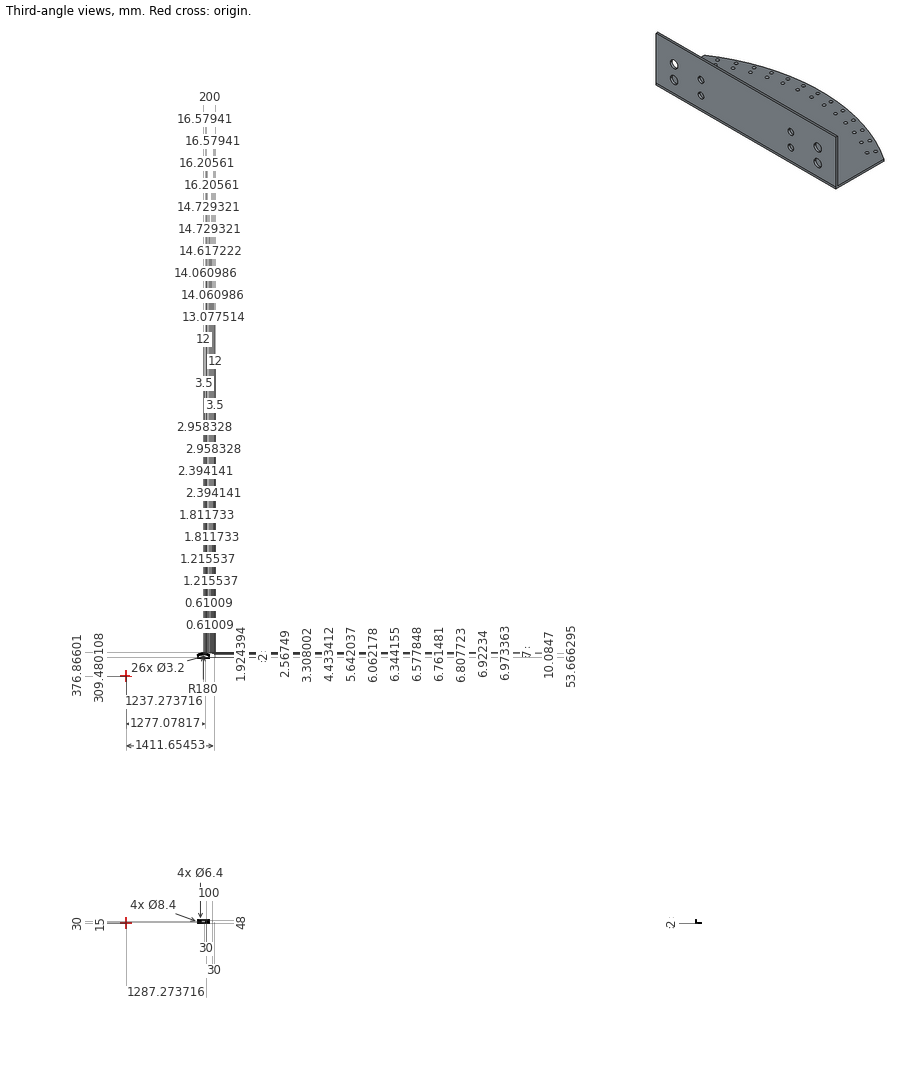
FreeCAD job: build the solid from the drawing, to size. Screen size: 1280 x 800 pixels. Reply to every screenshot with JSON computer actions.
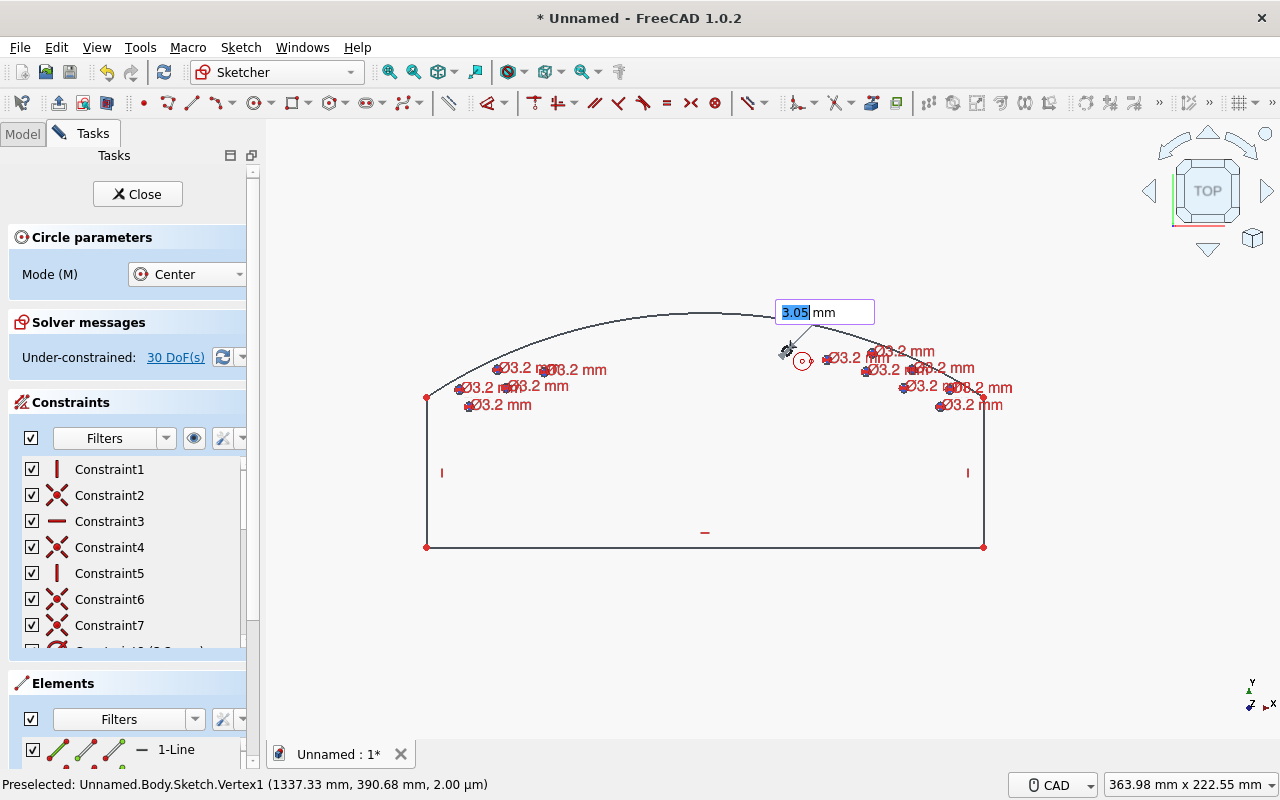
{"action": "type", "text": "3.2"}
{"action": "key", "text": "Return"}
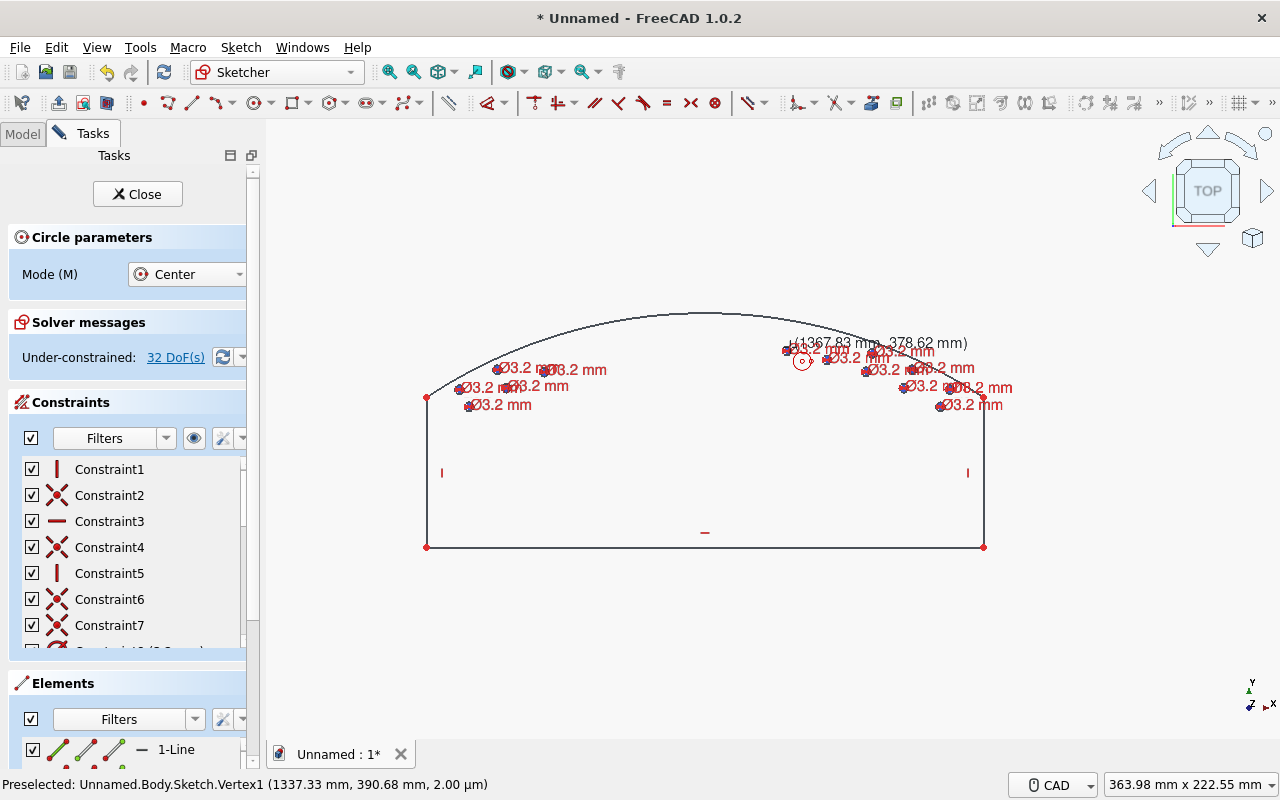
{"action": "scroll", "coordinate": [746, 345], "scroll_direction": "up", "scroll_amount": 9}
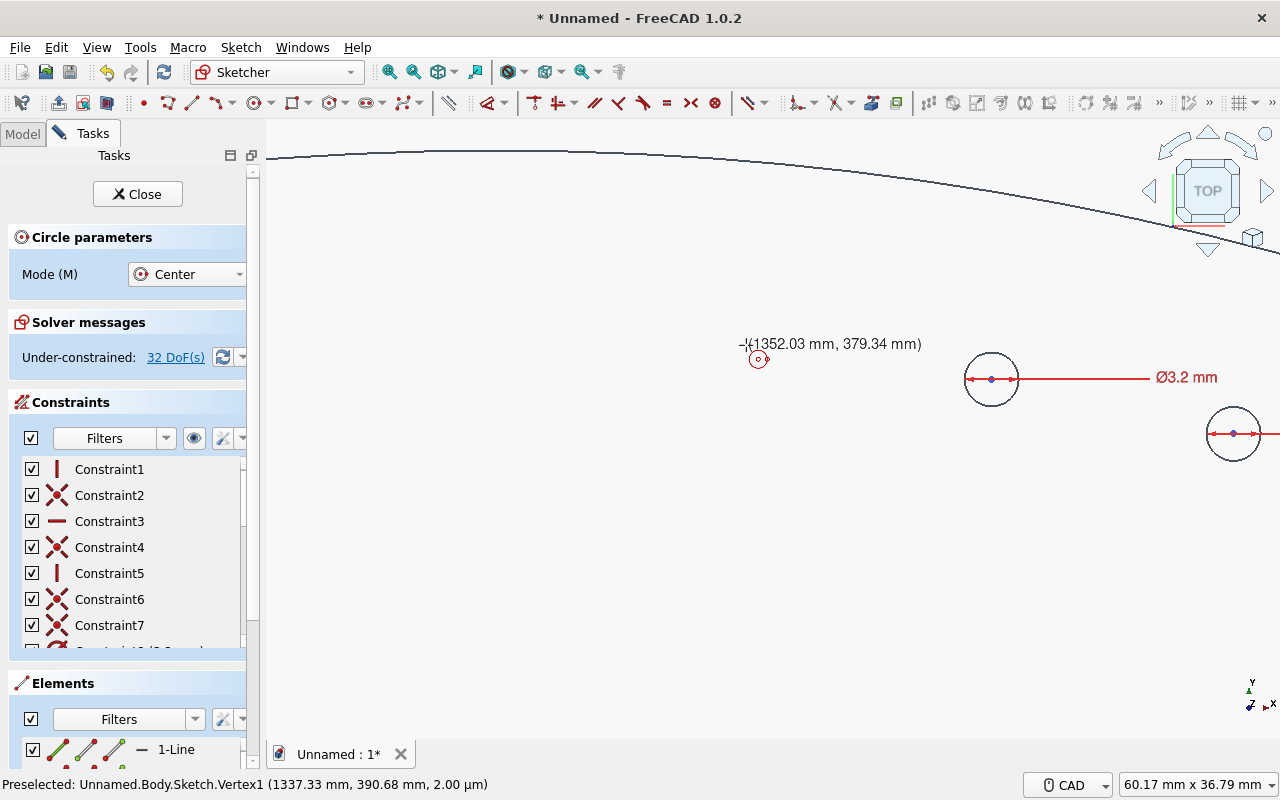
{"action": "scroll", "coordinate": [746, 345], "scroll_direction": "down", "scroll_amount": 9}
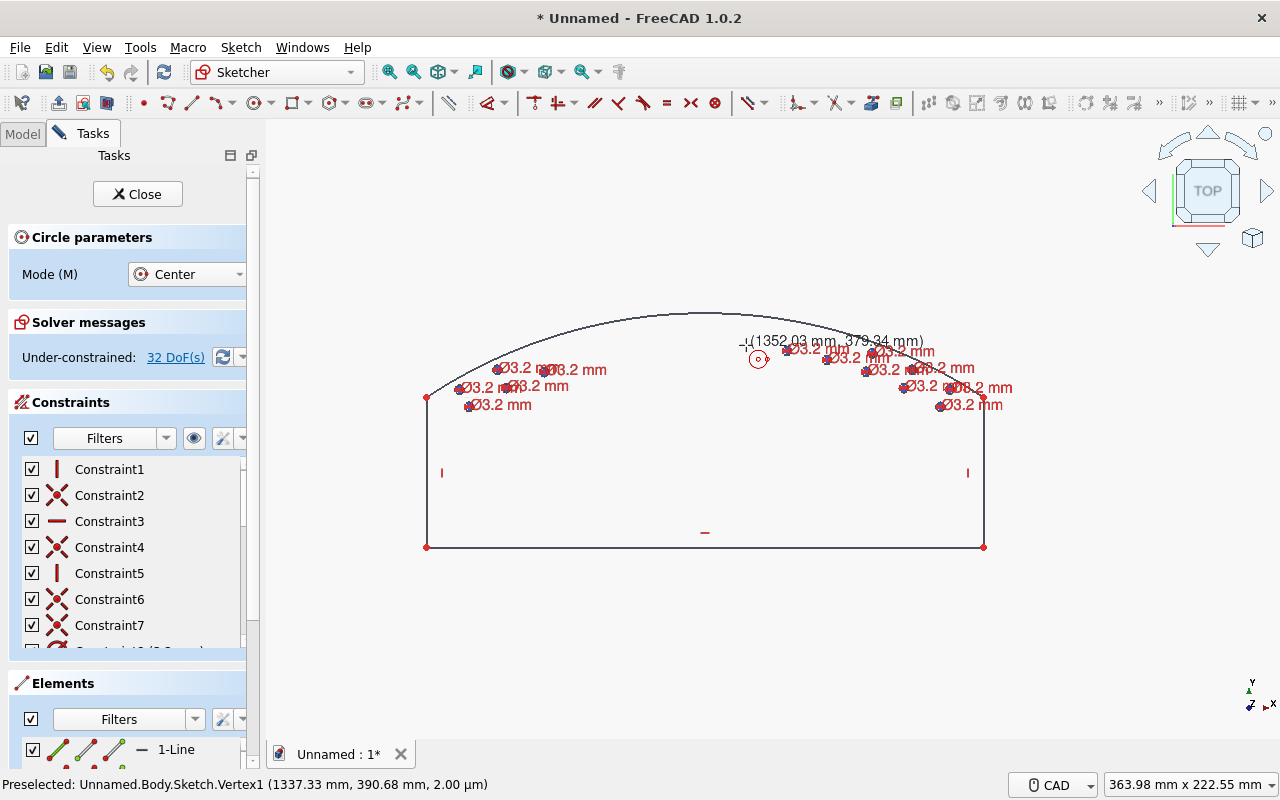
{"action": "left_click", "coordinate": [746, 345]}
{"action": "mouse_move", "coordinate": [749, 341]}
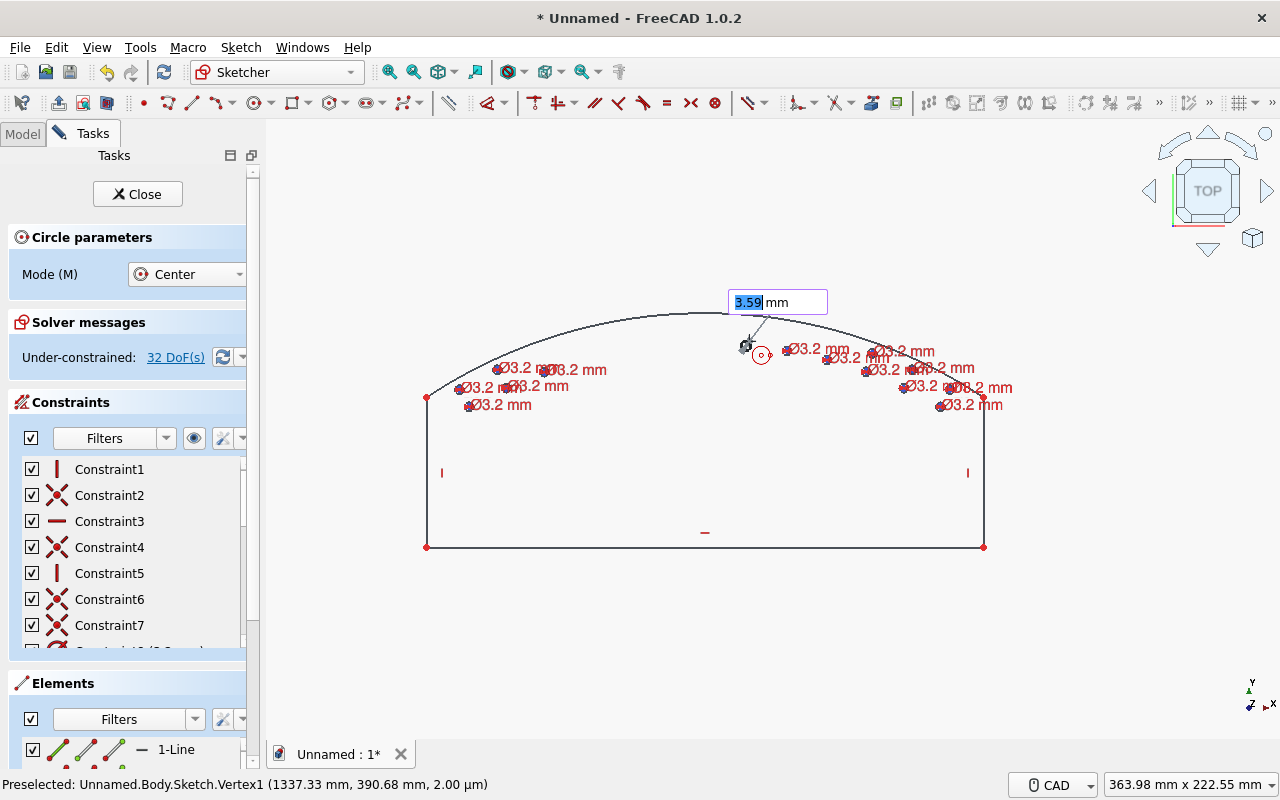
{"action": "type", "text": "3.2"}
{"action": "key", "text": "Return"}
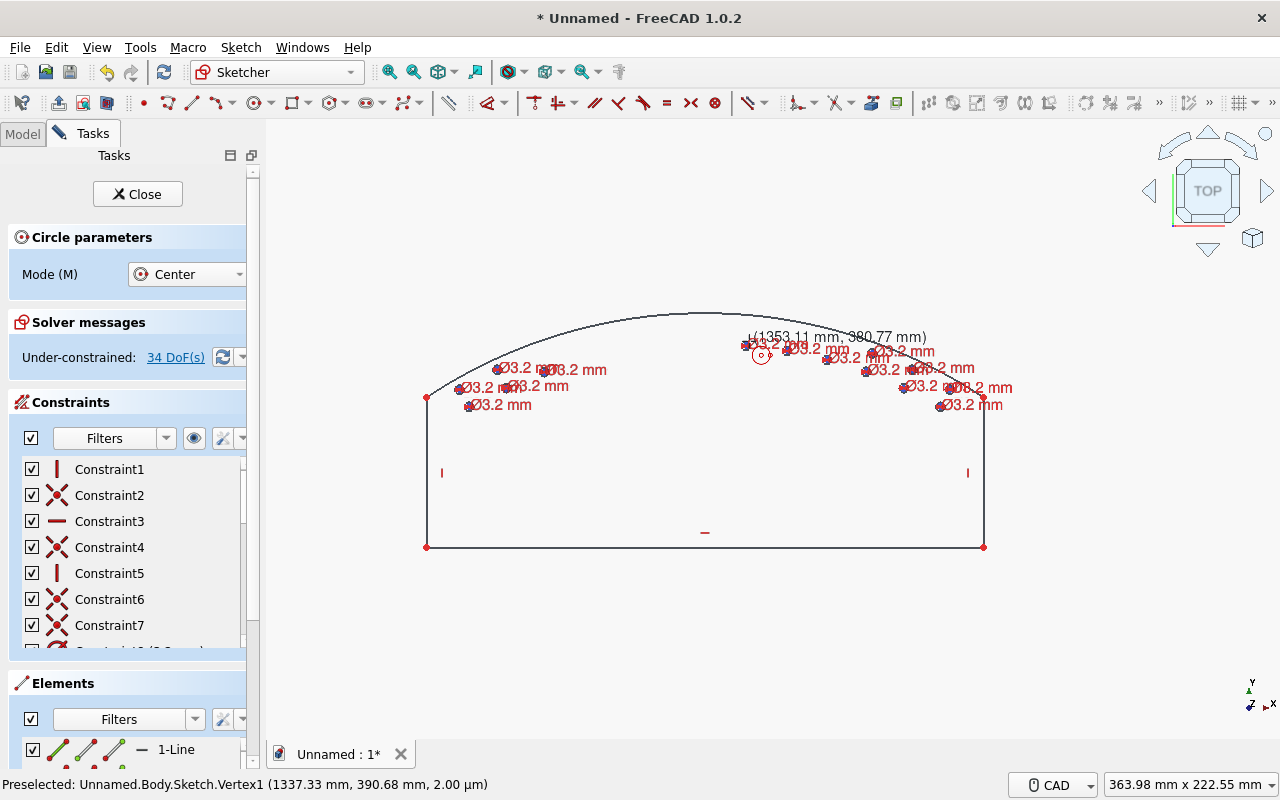
{"action": "scroll", "coordinate": [705, 343], "scroll_direction": "up", "scroll_amount": 9}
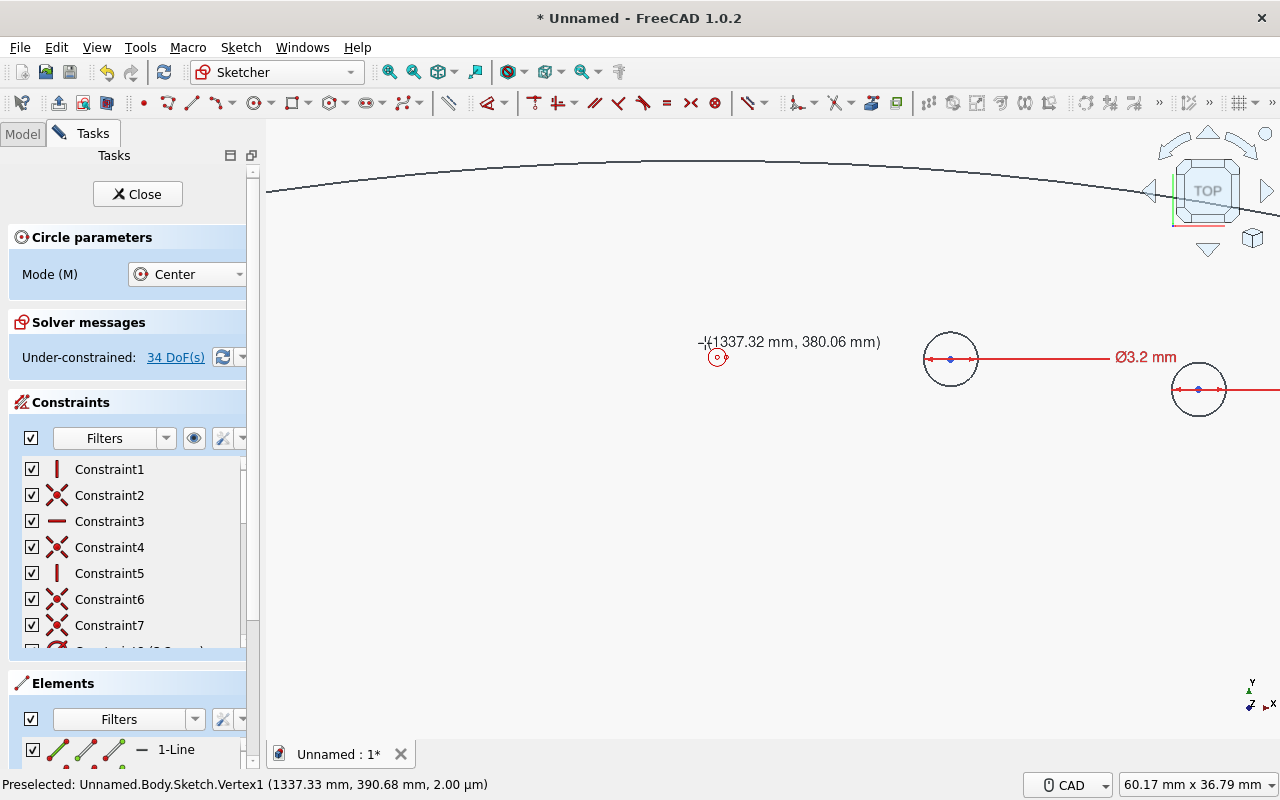
{"action": "scroll", "coordinate": [705, 343], "scroll_direction": "down", "scroll_amount": 9}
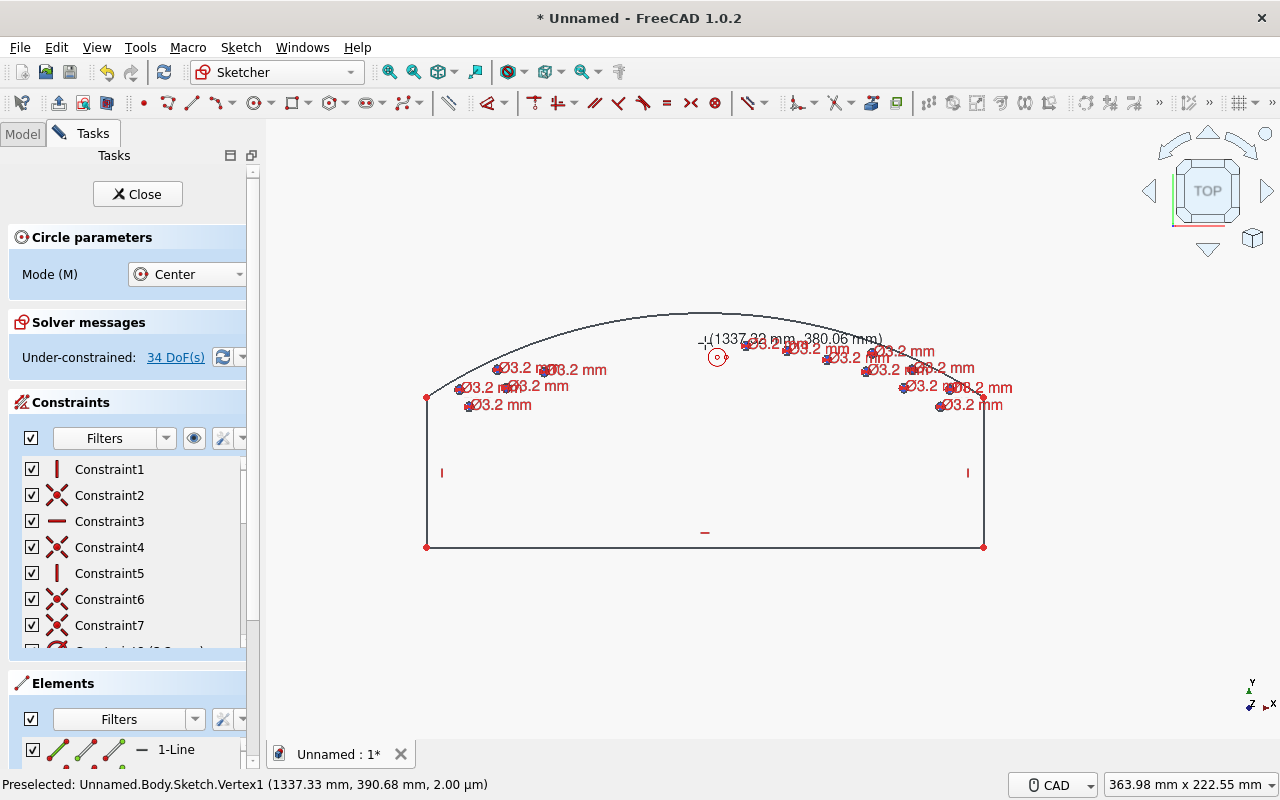
{"action": "left_click", "coordinate": [705, 343]}
{"action": "mouse_move", "coordinate": [708, 340]}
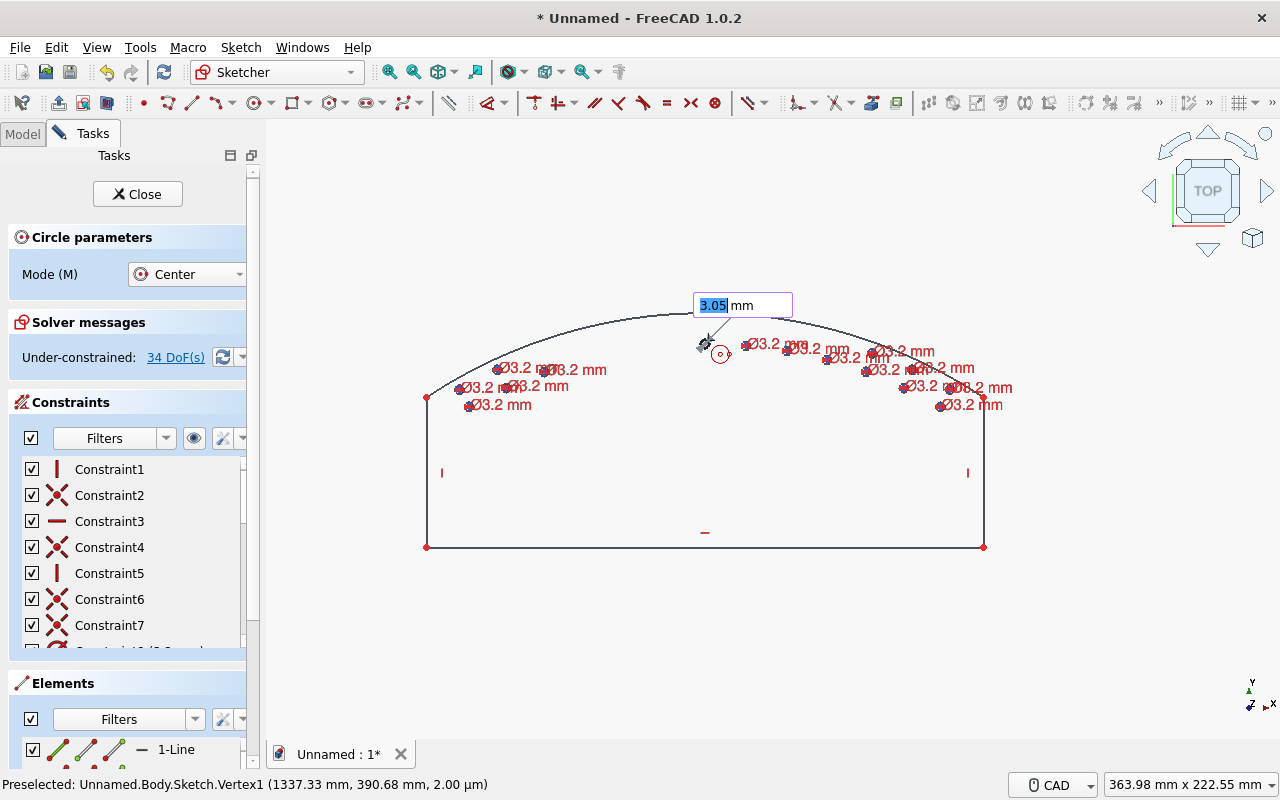
{"action": "type", "text": "3.2"}
{"action": "key", "text": "Return"}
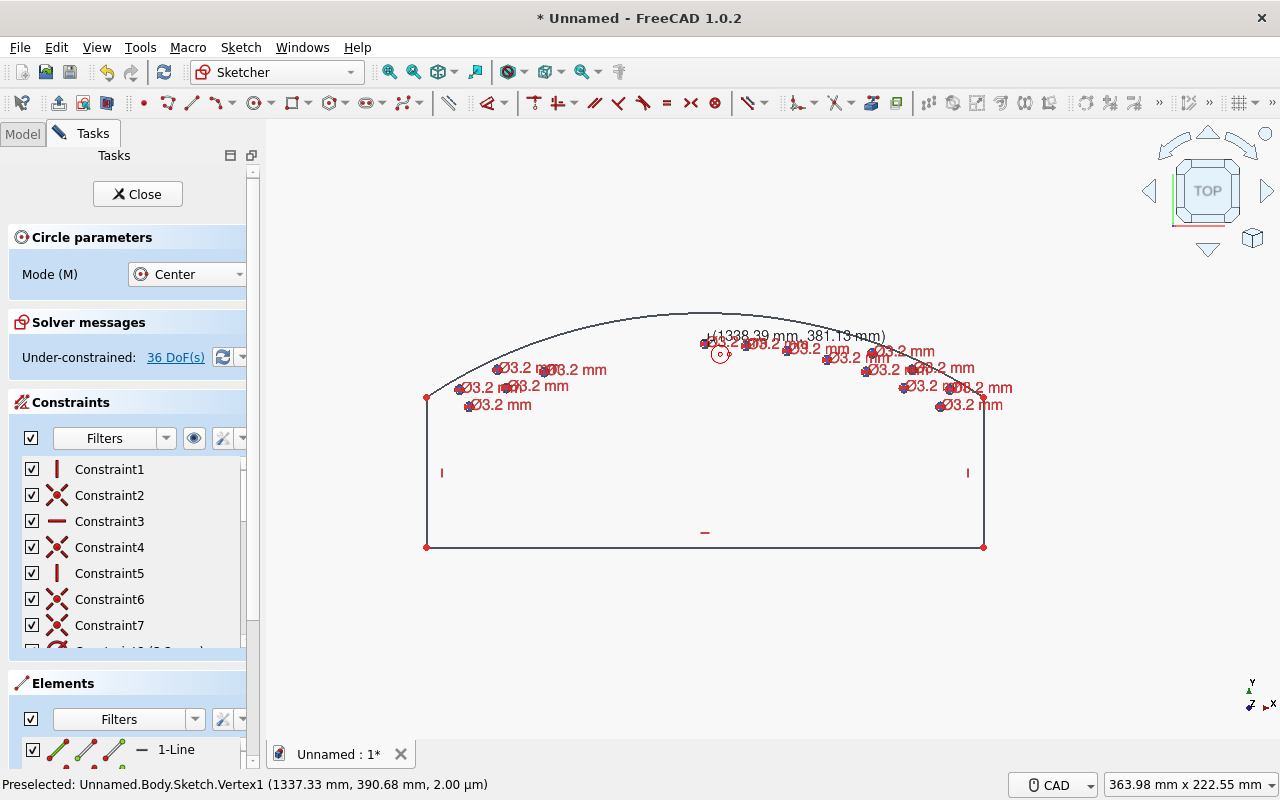
{"action": "scroll", "coordinate": [832, 340], "scroll_direction": "up", "scroll_amount": 9}